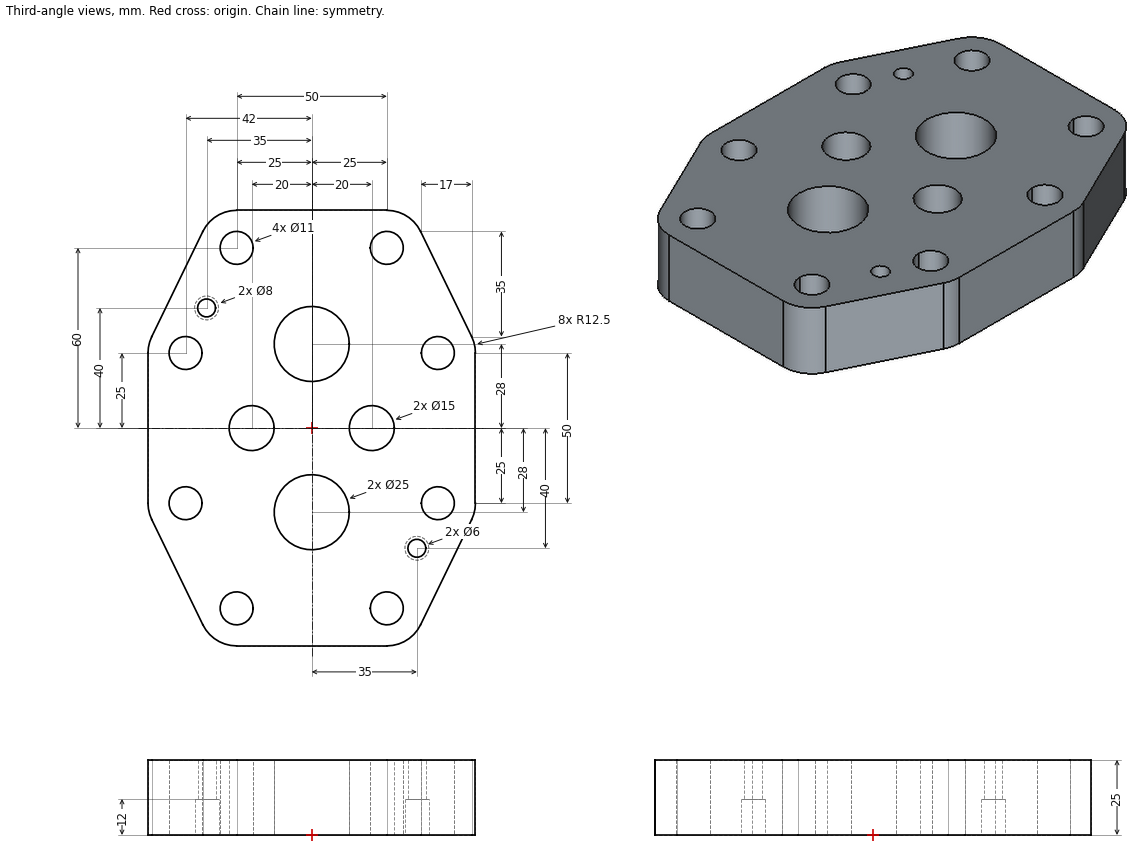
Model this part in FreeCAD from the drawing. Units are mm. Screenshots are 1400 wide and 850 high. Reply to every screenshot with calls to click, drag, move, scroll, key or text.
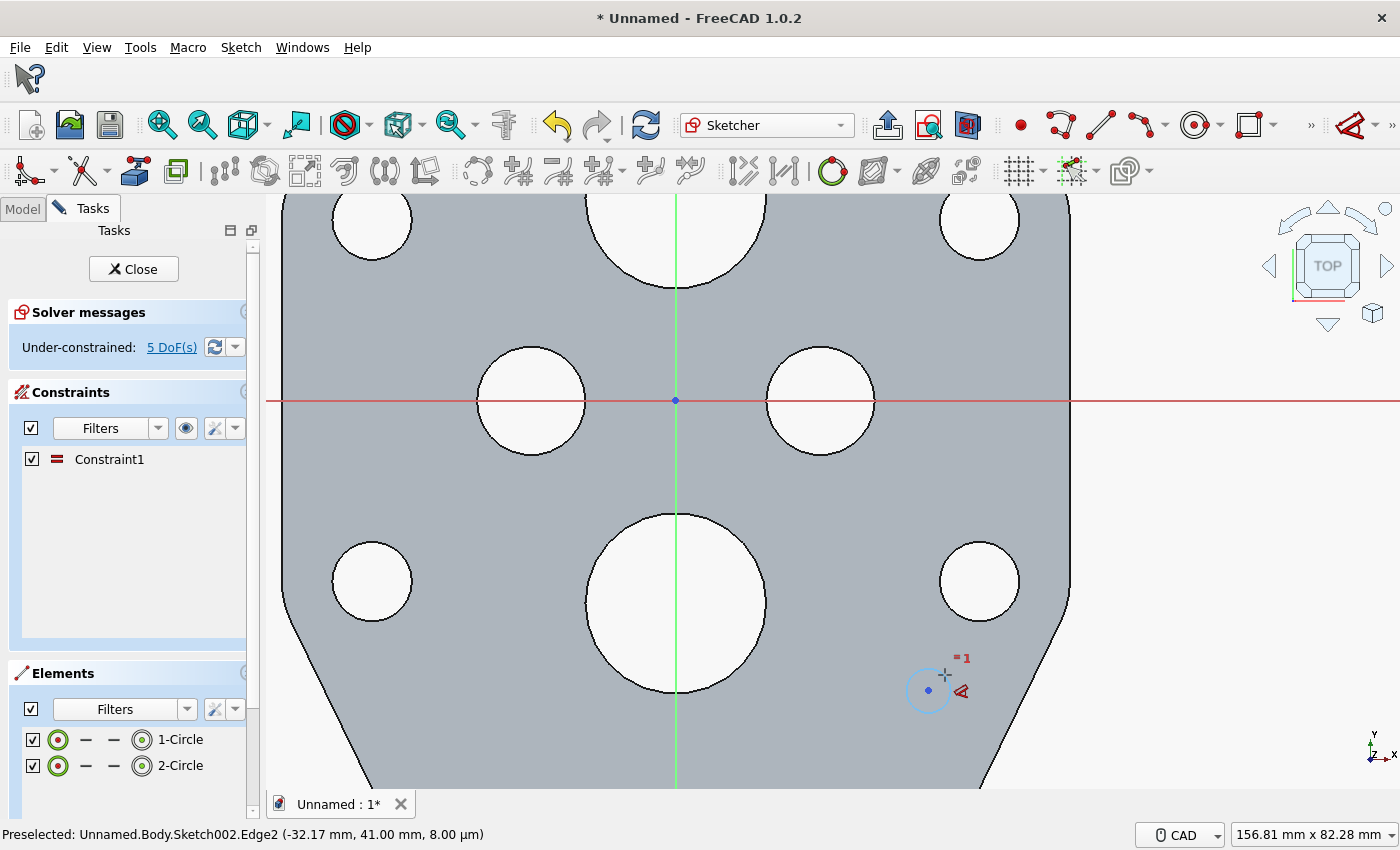
click(944, 675)
click(966, 652)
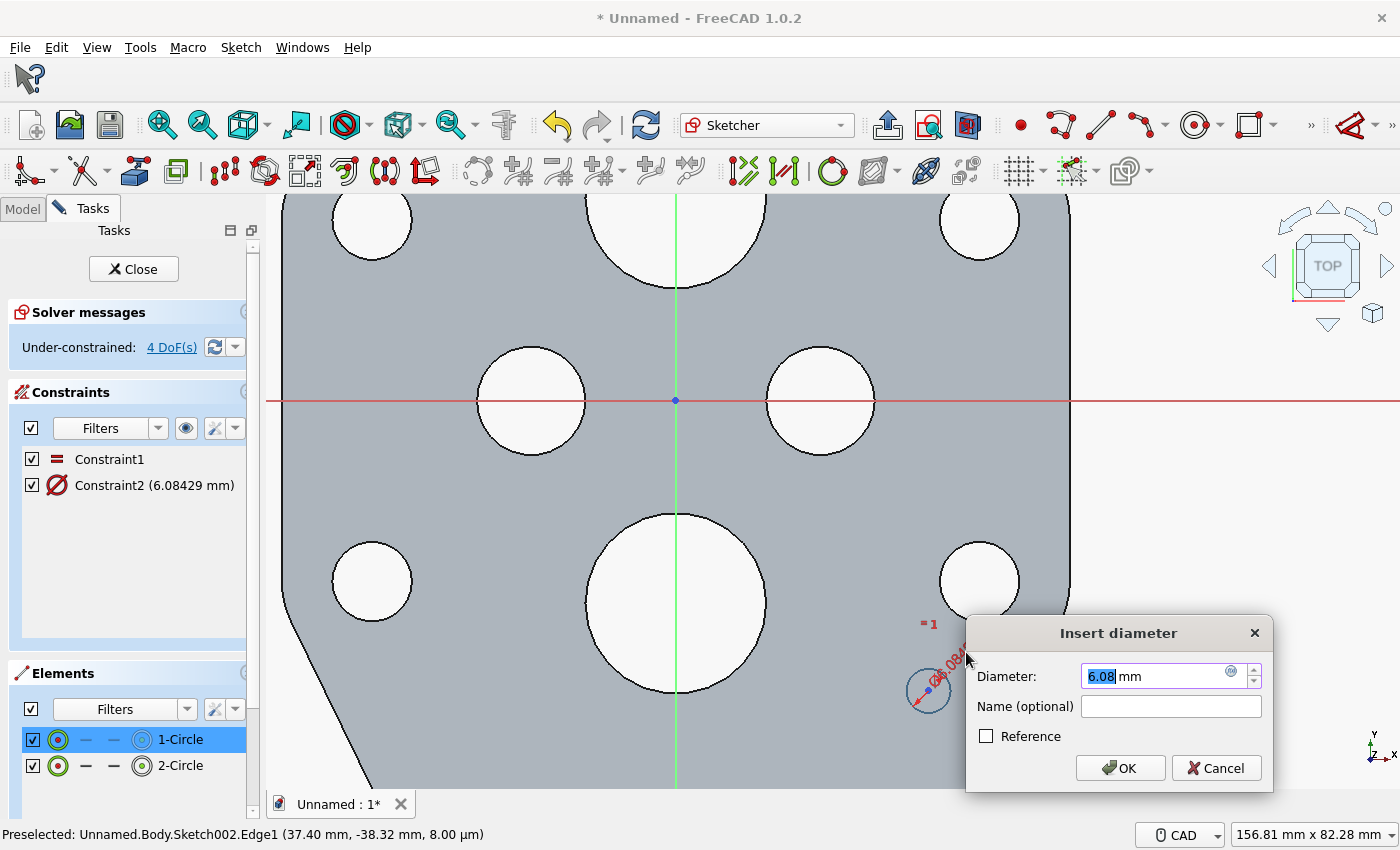
text(6)
key(Return)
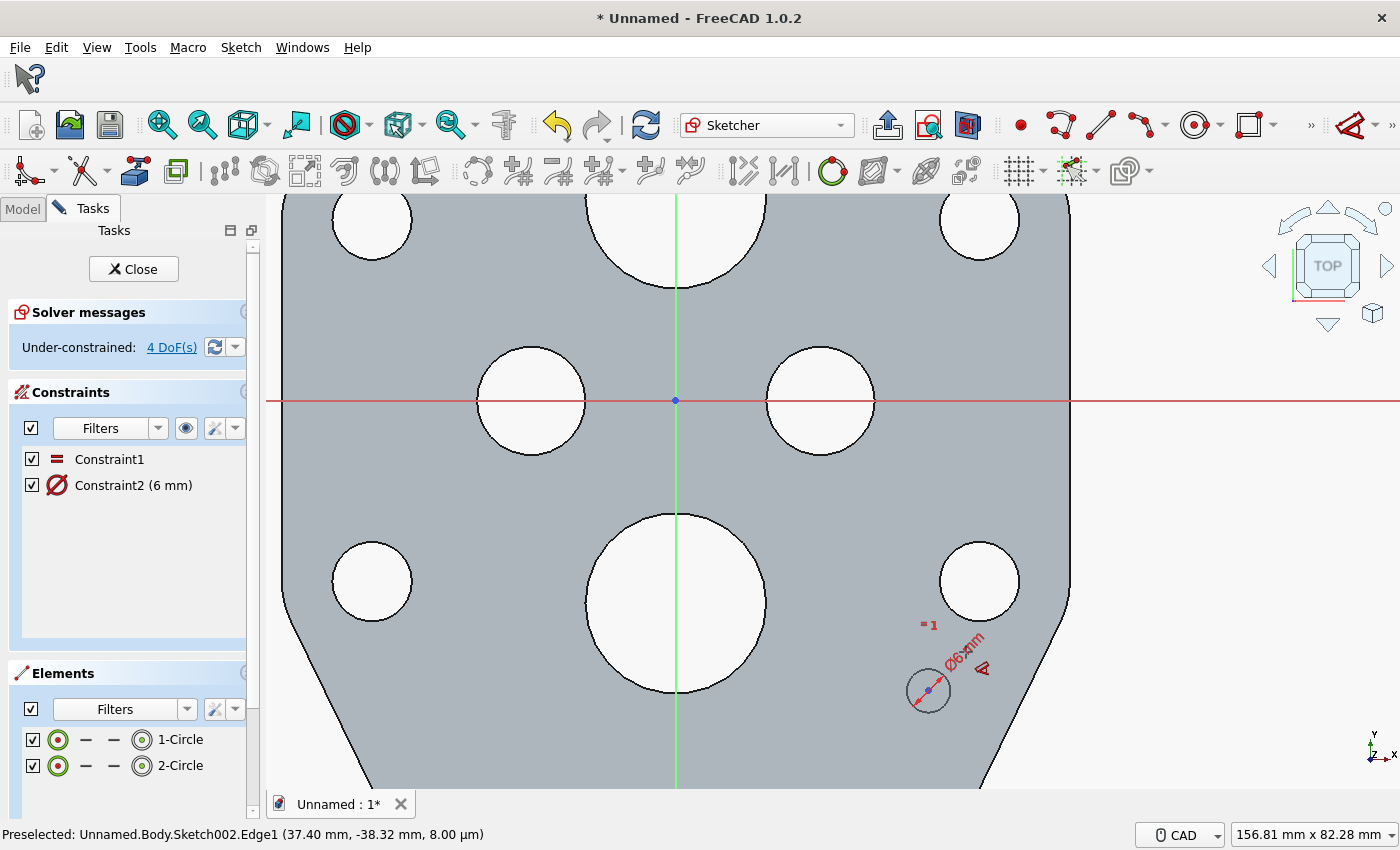
click(929, 691)
click(802, 725)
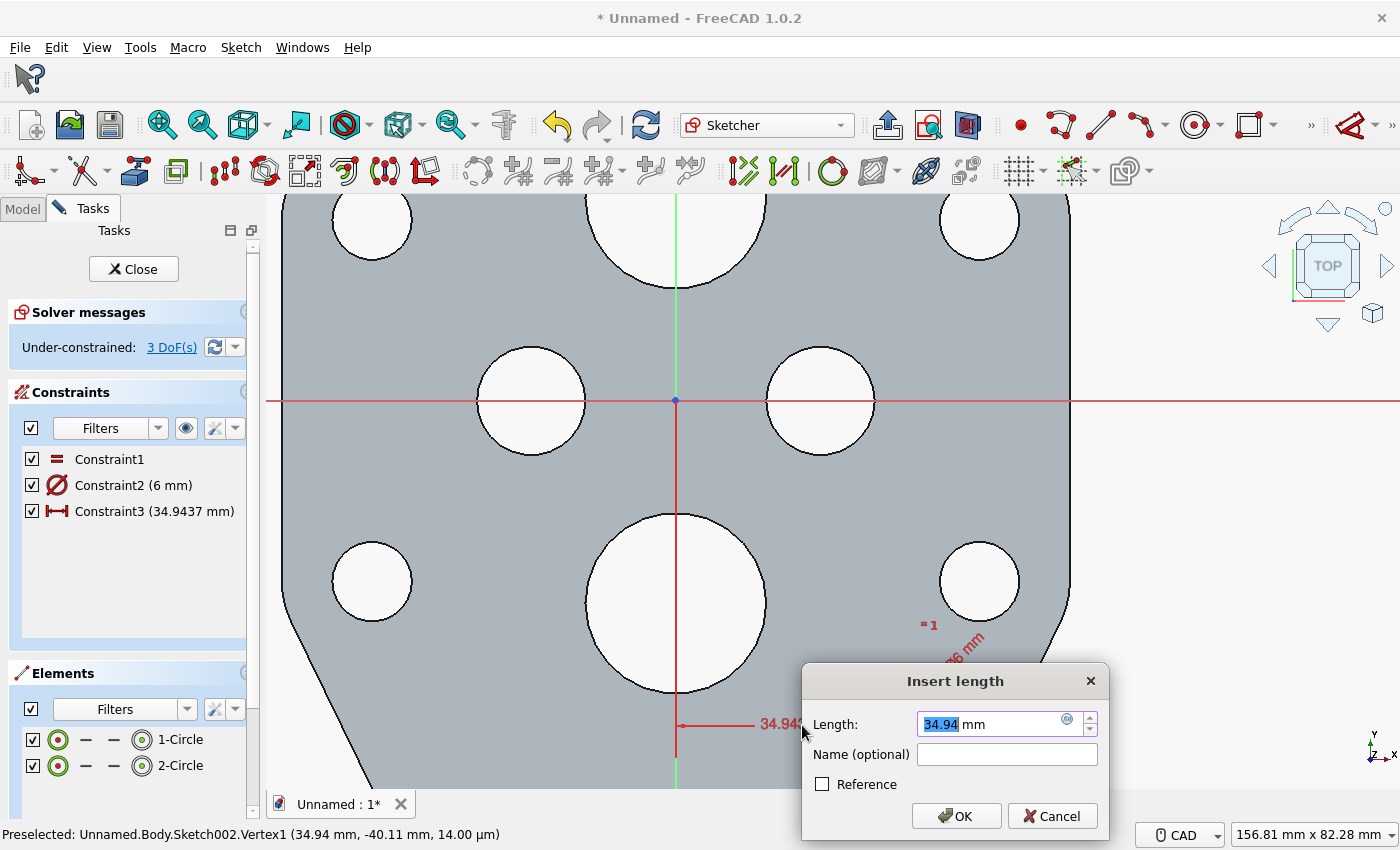
text(35)
key(Return)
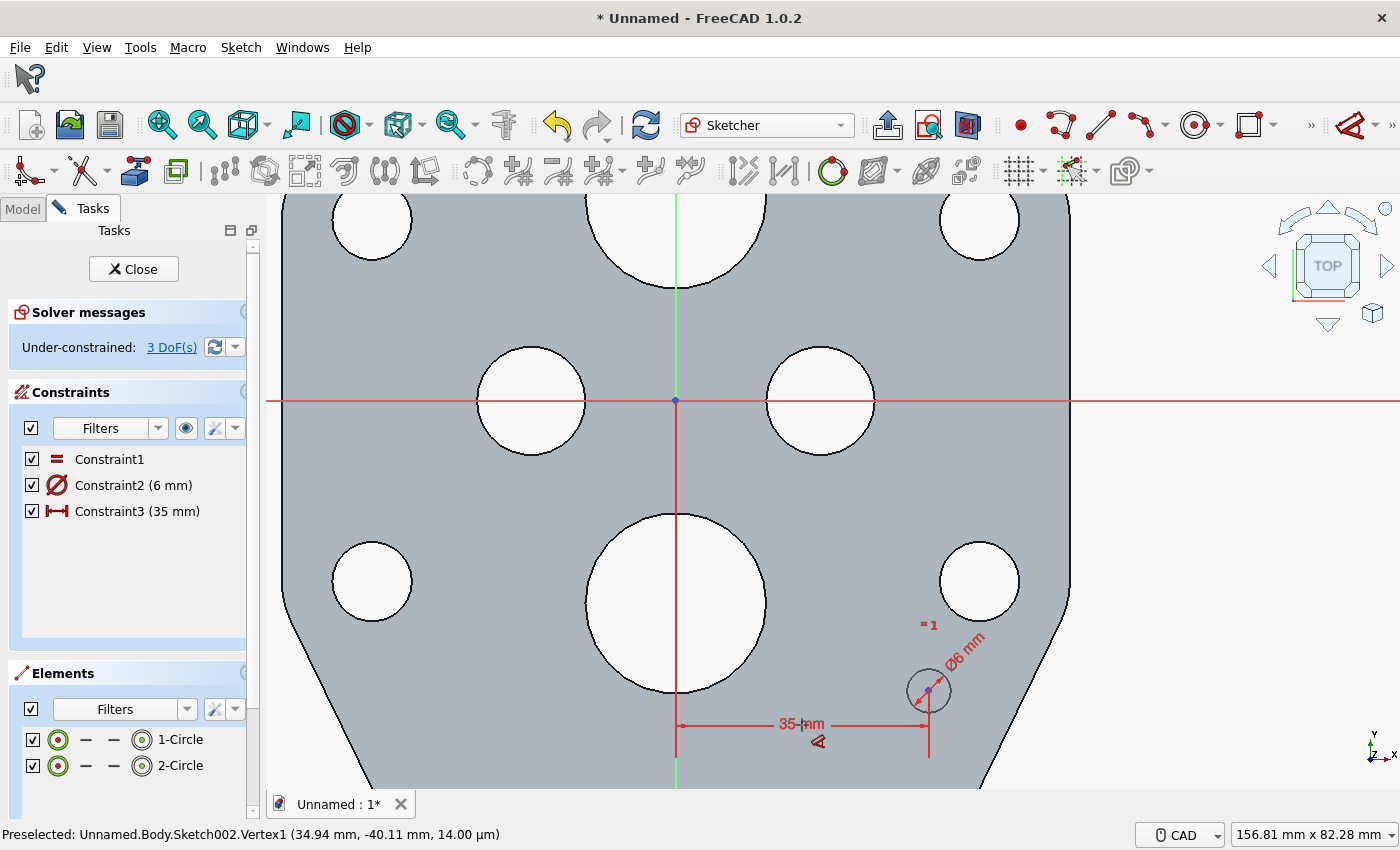
click(929, 691)
click(963, 546)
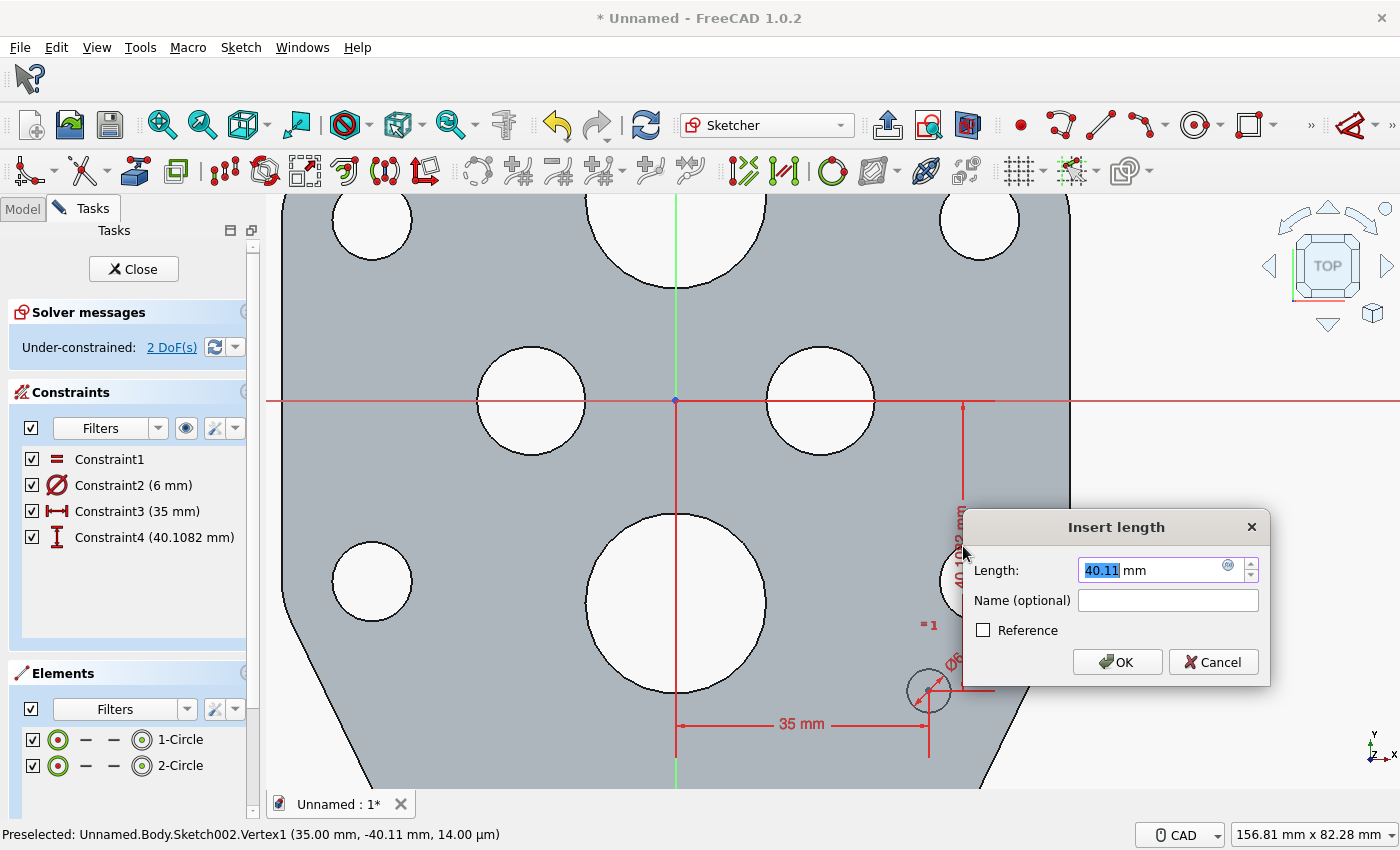
text(40)
key(Return)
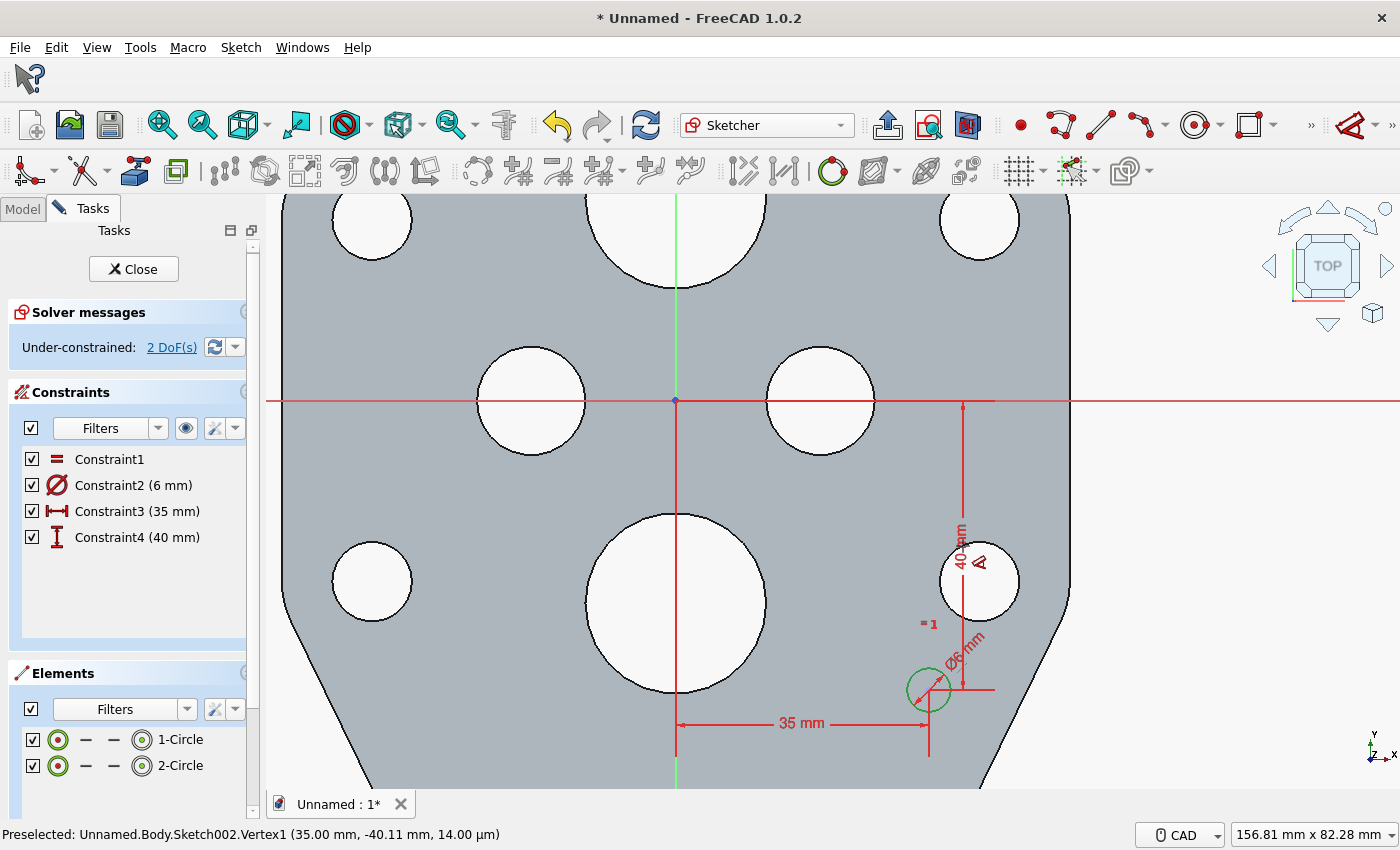
scroll(945, 676, down, 2)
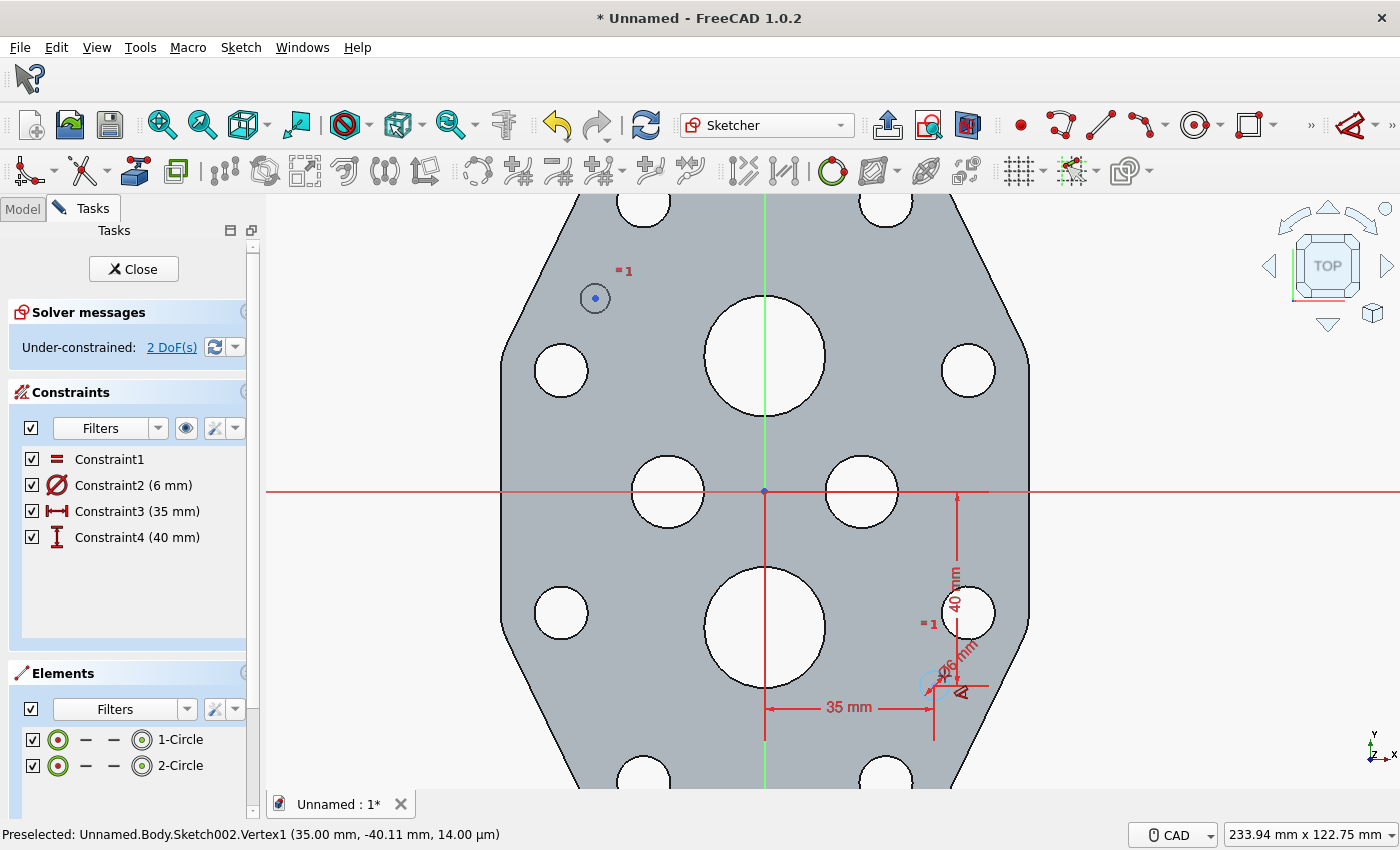
click(595, 299)
click(680, 265)